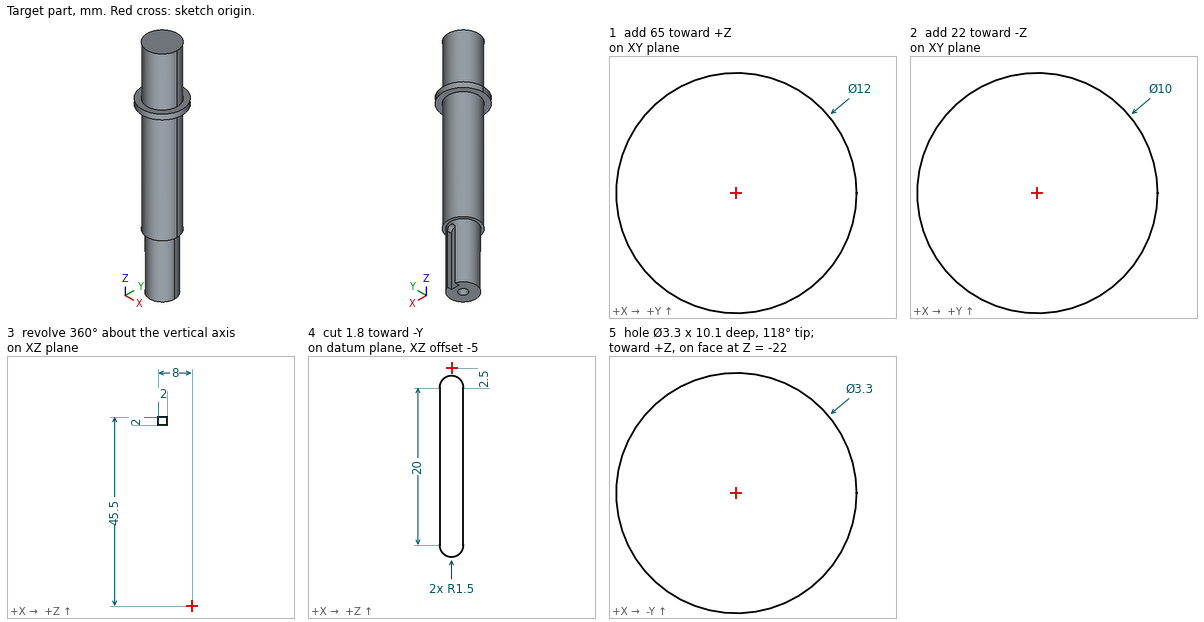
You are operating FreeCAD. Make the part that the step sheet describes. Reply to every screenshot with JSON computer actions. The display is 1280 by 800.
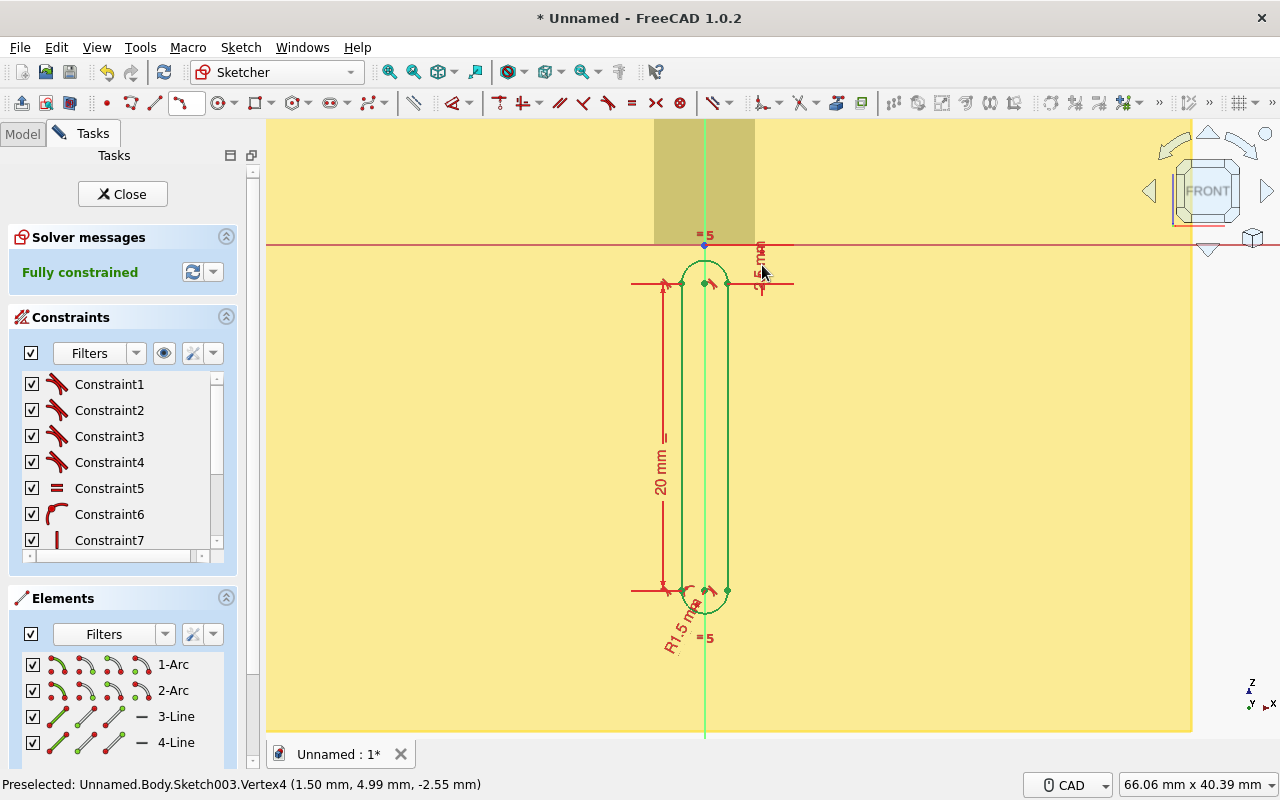
{"action": "left_click", "coordinate": [123, 194]}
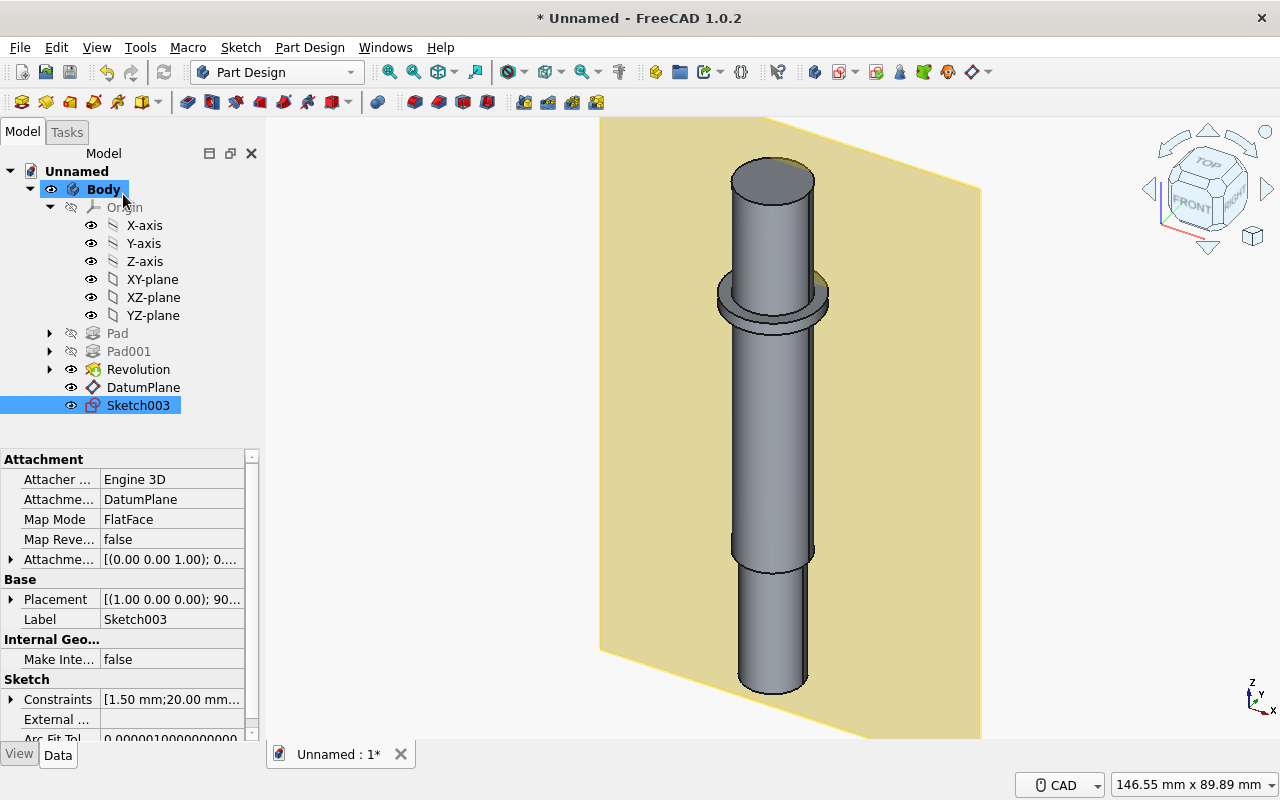
{"action": "left_click", "coordinate": [188, 102]}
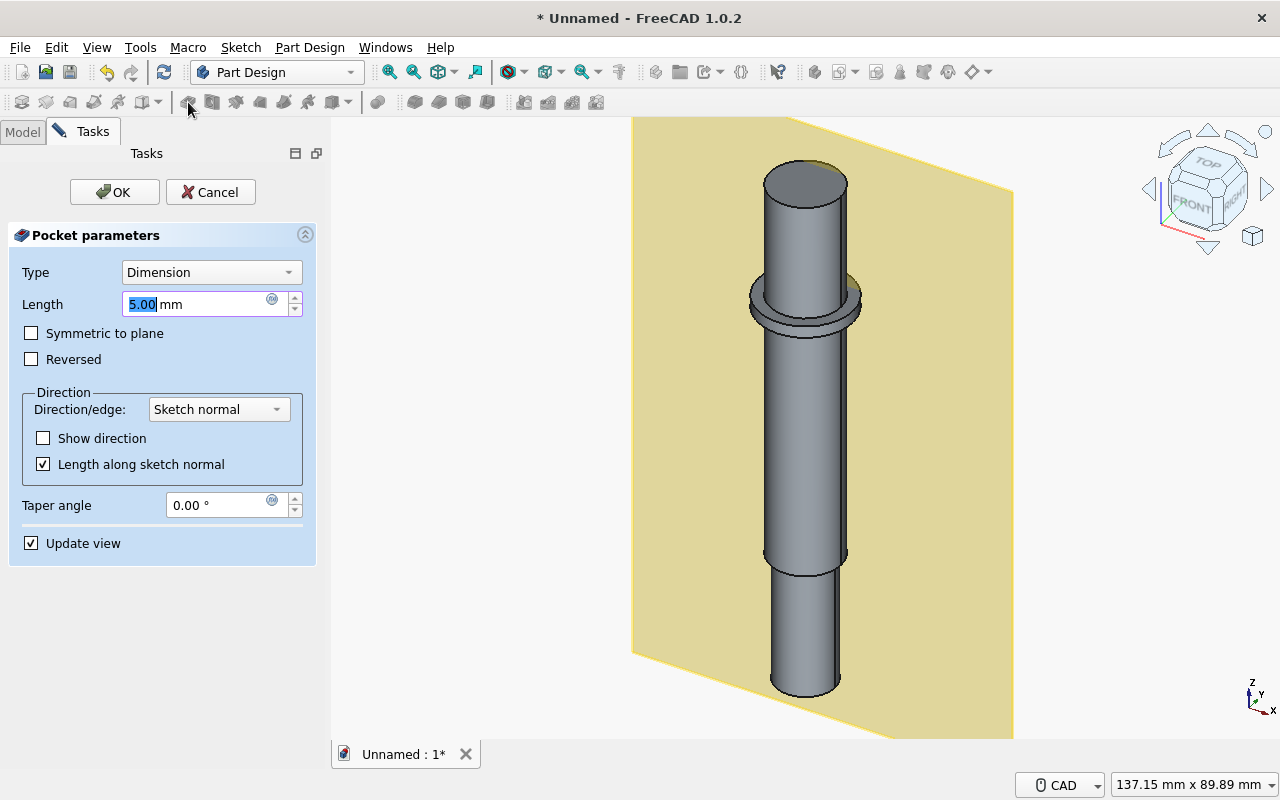
{"action": "type", "text": "1.8"}
{"action": "key", "text": "Tab"}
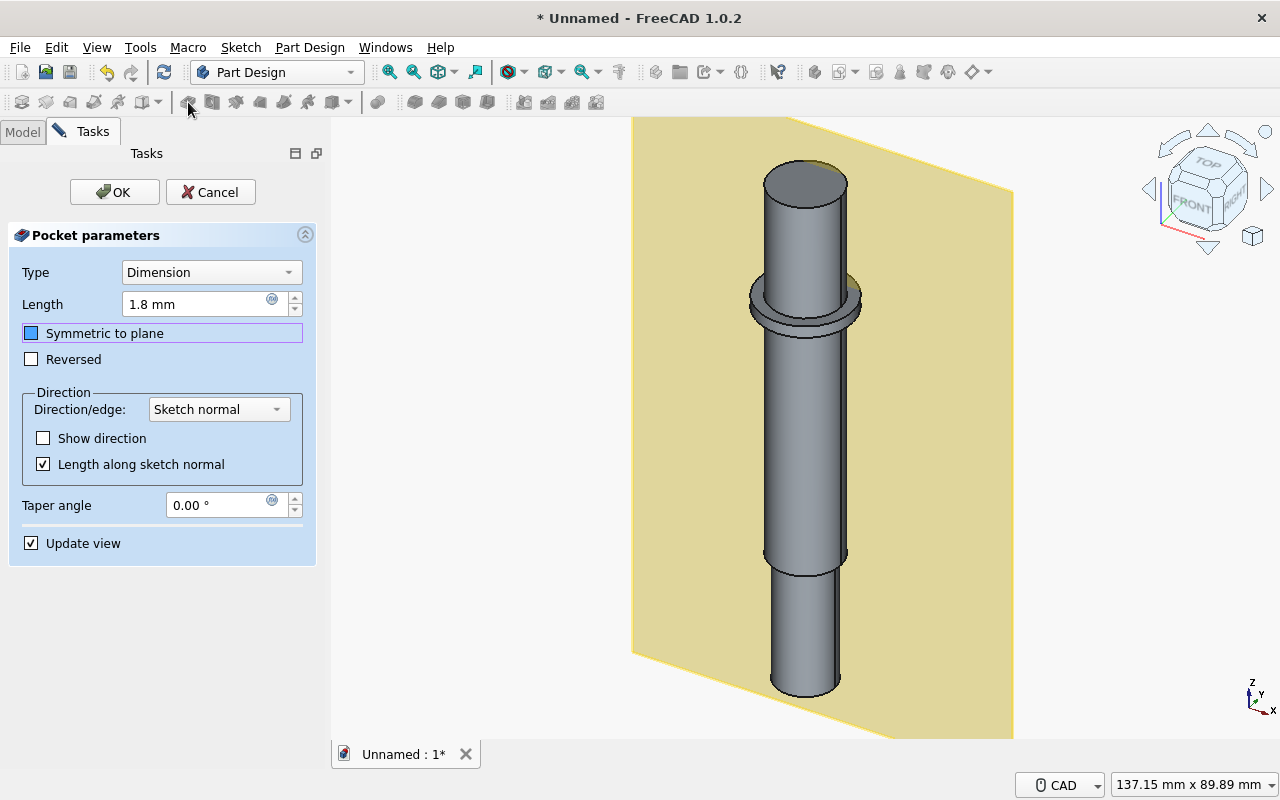
{"action": "left_click", "coordinate": [30, 359]}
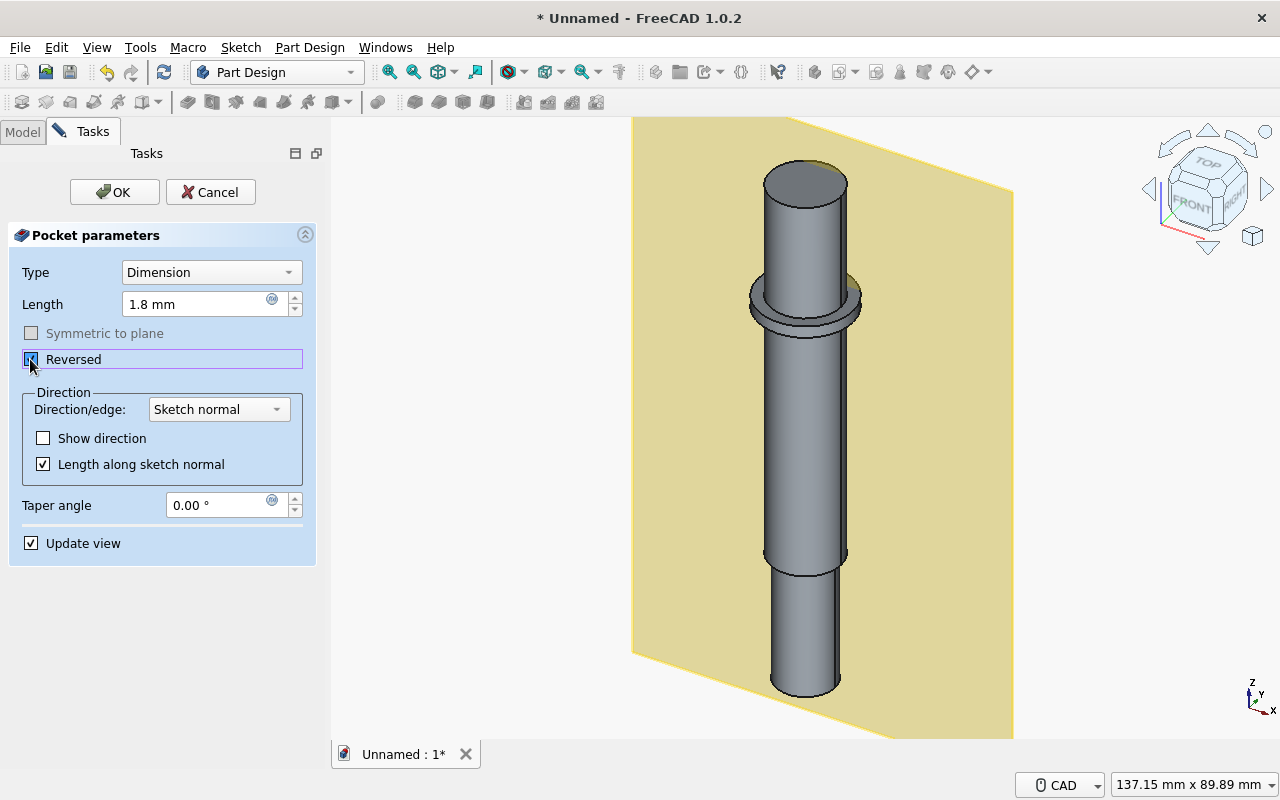
{"action": "left_click", "coordinate": [115, 192]}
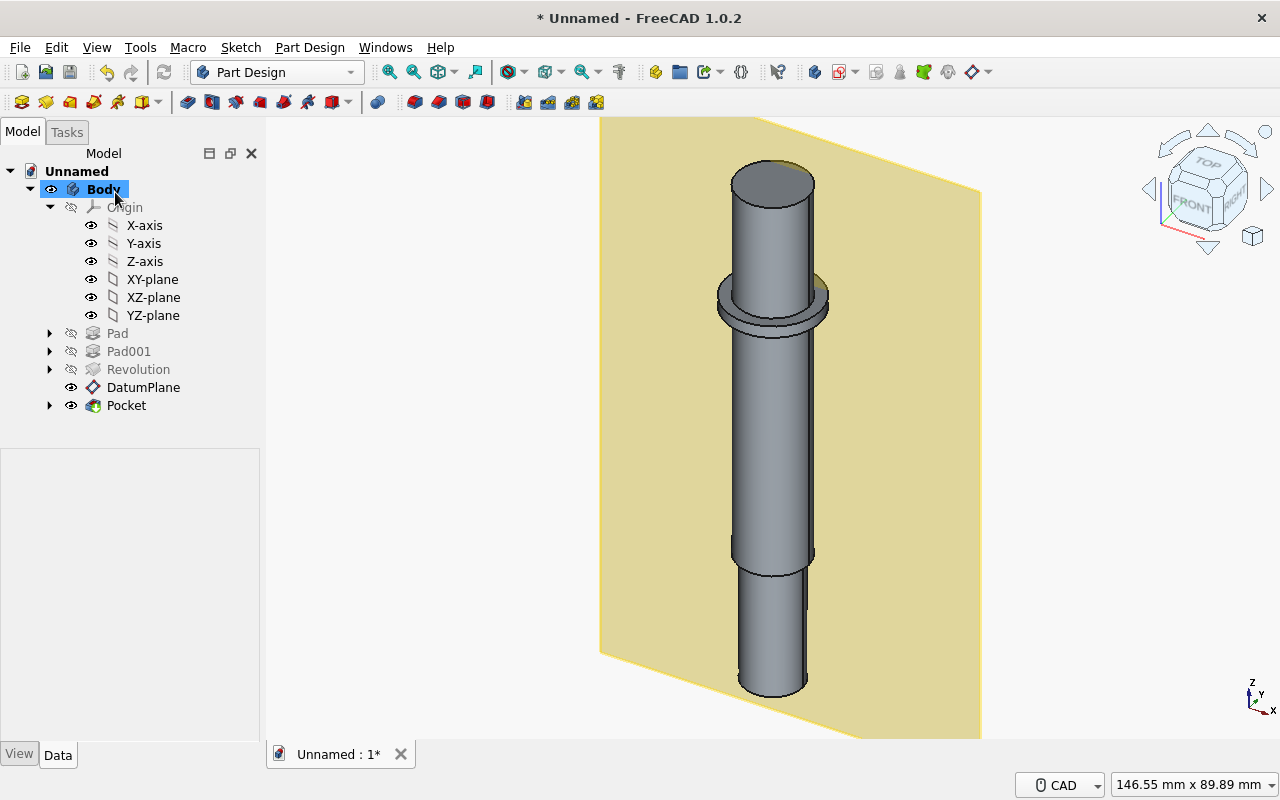
{"action": "left_click", "coordinate": [116, 387]}
{"action": "key", "text": "space"}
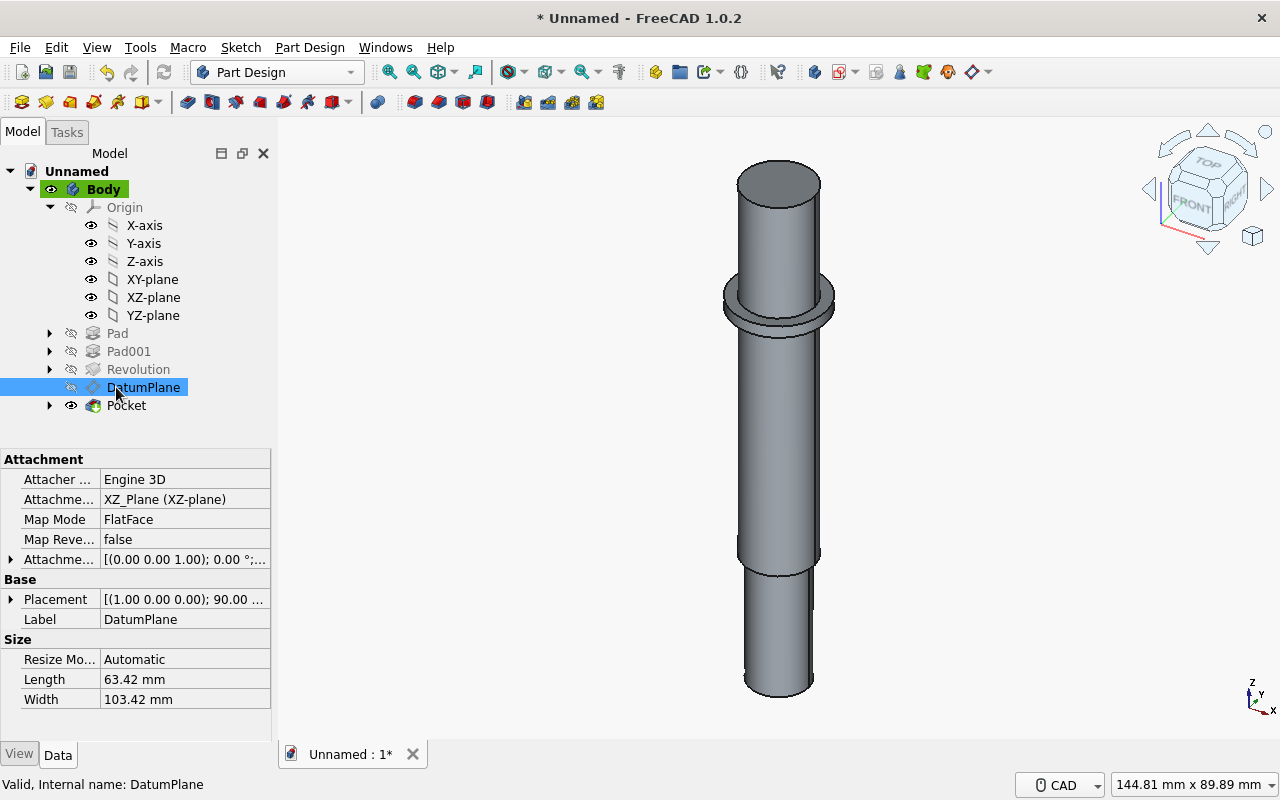
{"action": "key", "text": "5"}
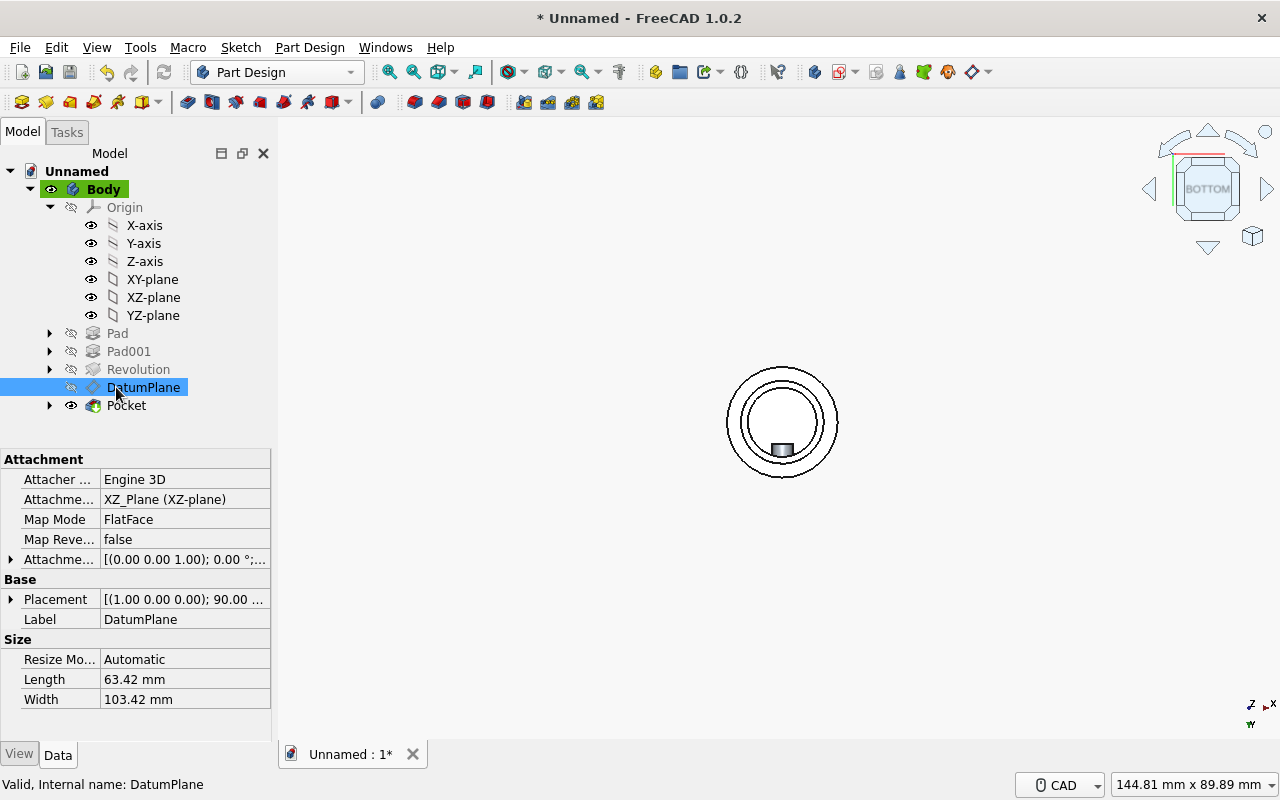
{"action": "left_click", "coordinate": [390, 72]}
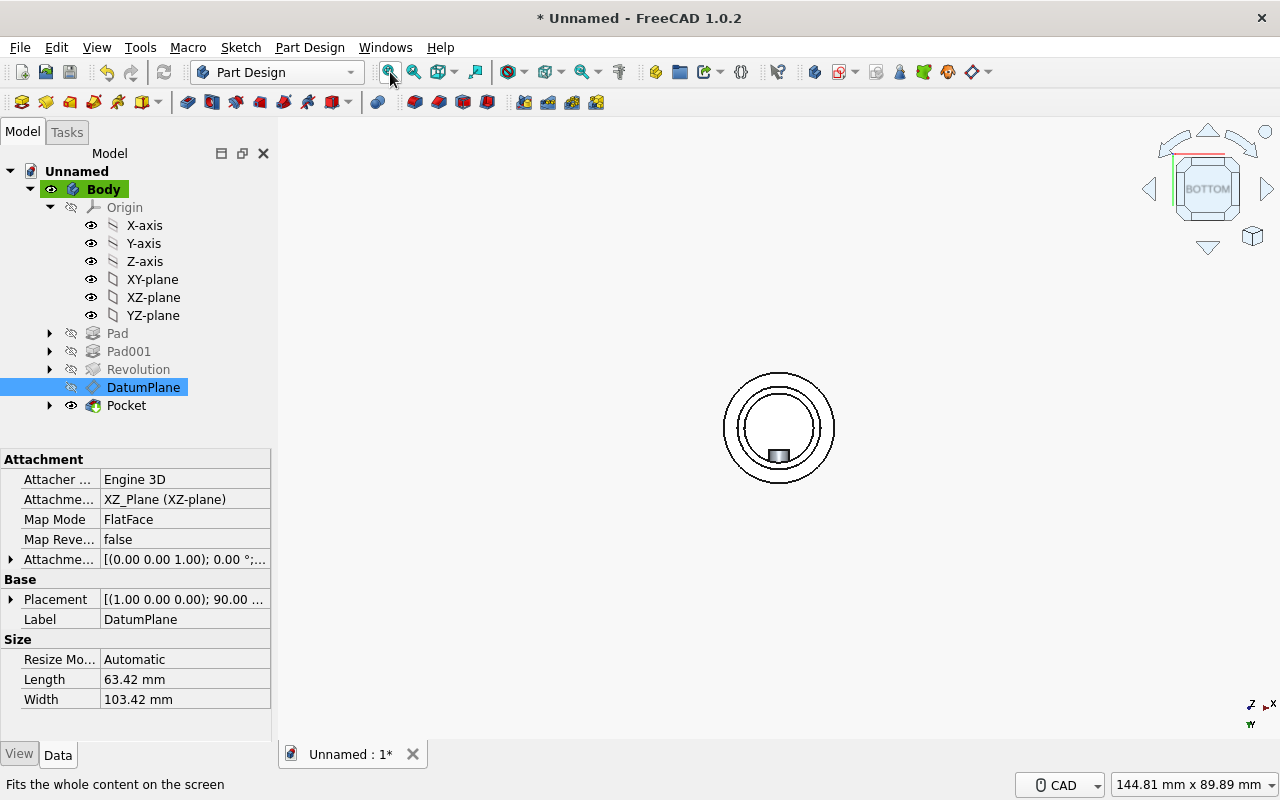
{"action": "left_click", "coordinate": [779, 417]}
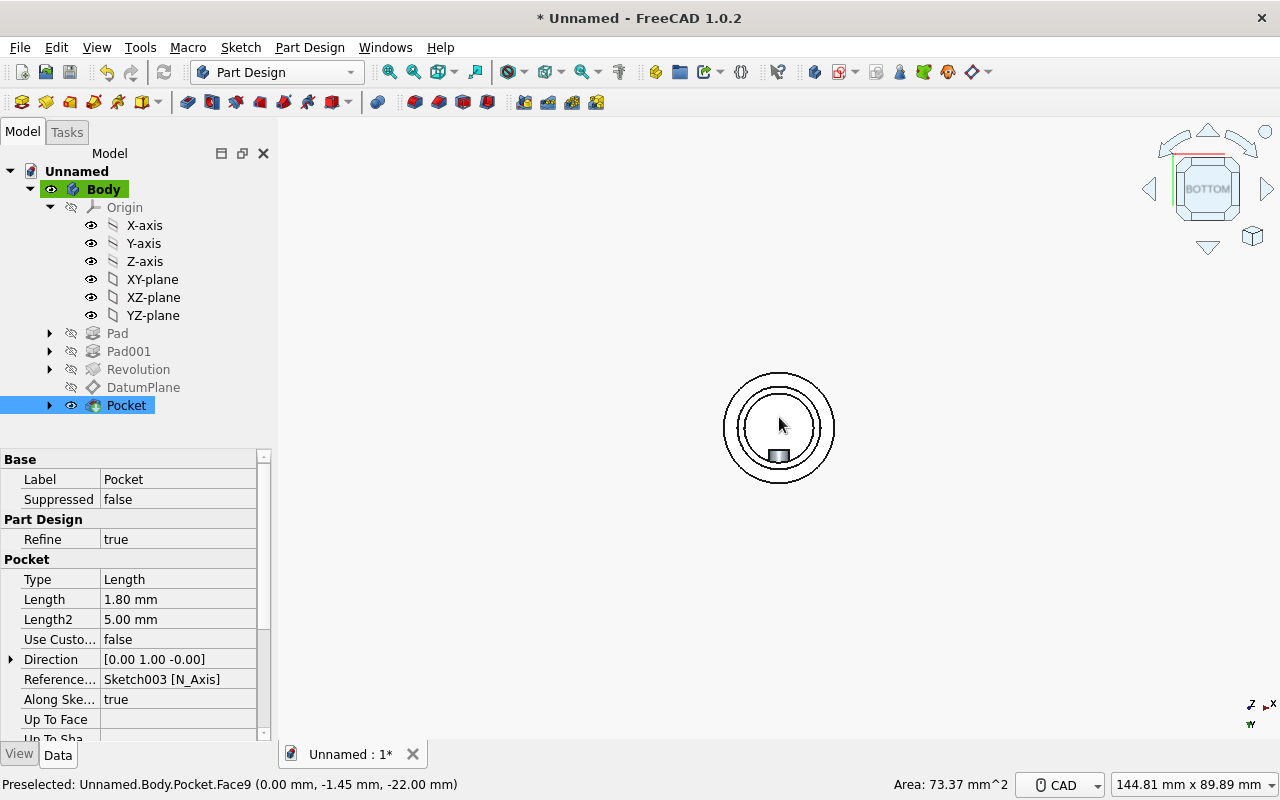
{"action": "left_click", "coordinate": [840, 72]}